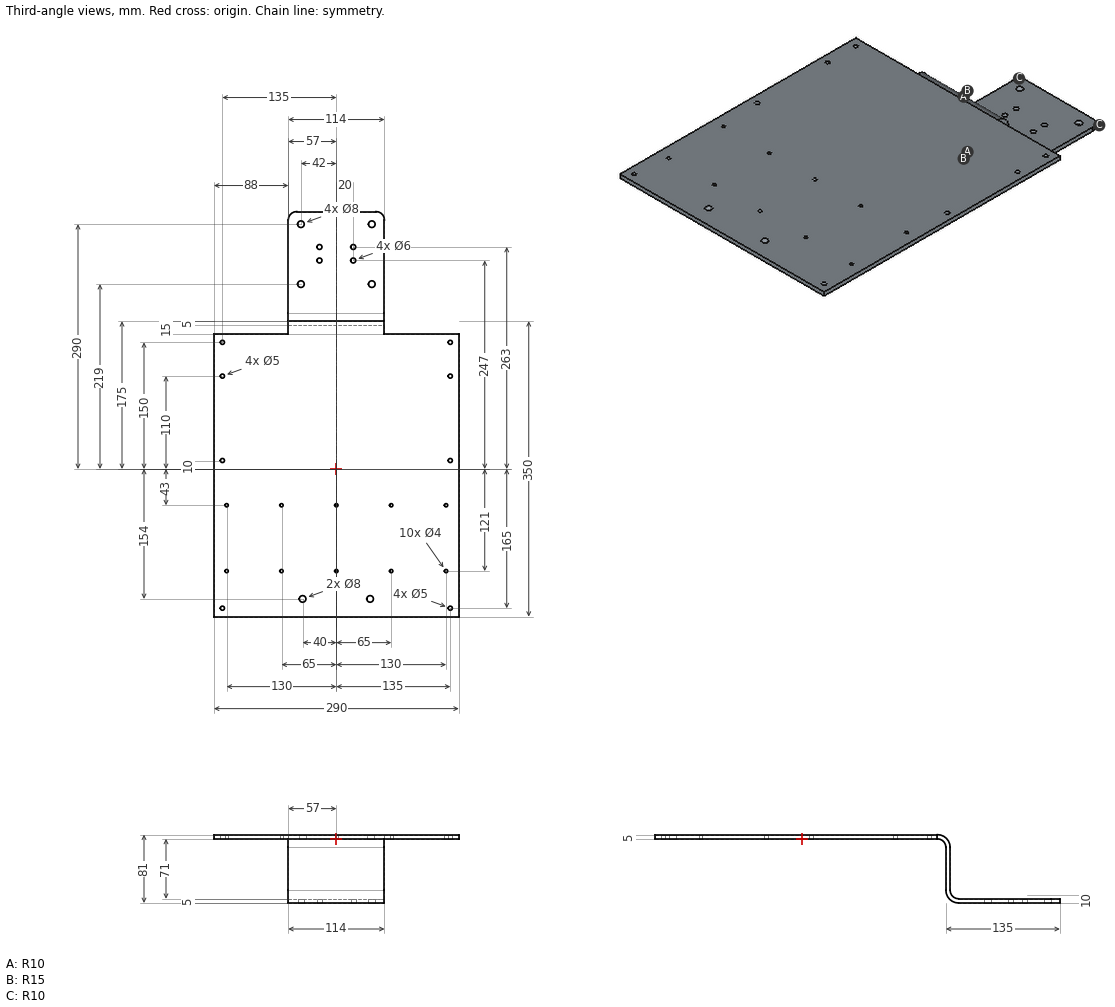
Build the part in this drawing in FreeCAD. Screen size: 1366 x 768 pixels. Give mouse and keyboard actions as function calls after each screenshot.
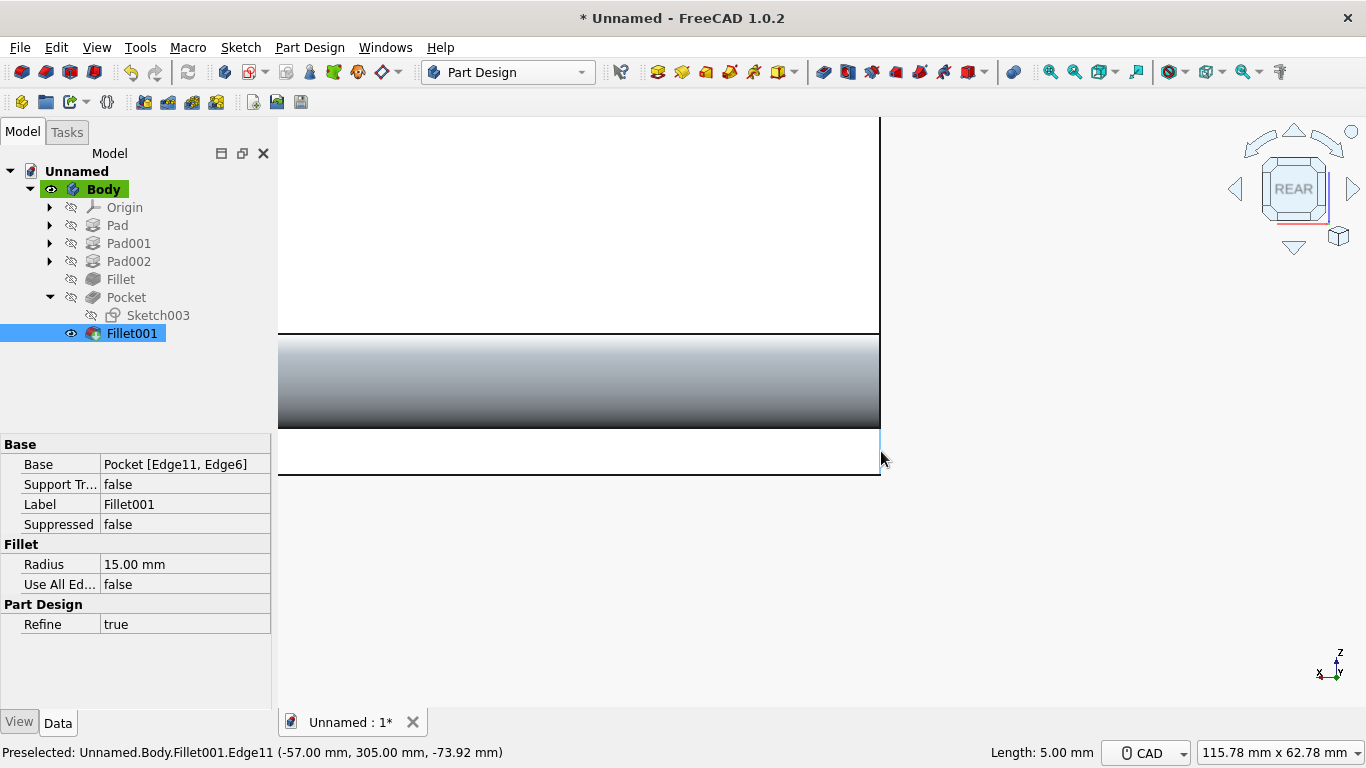
click(880, 451, ctrl)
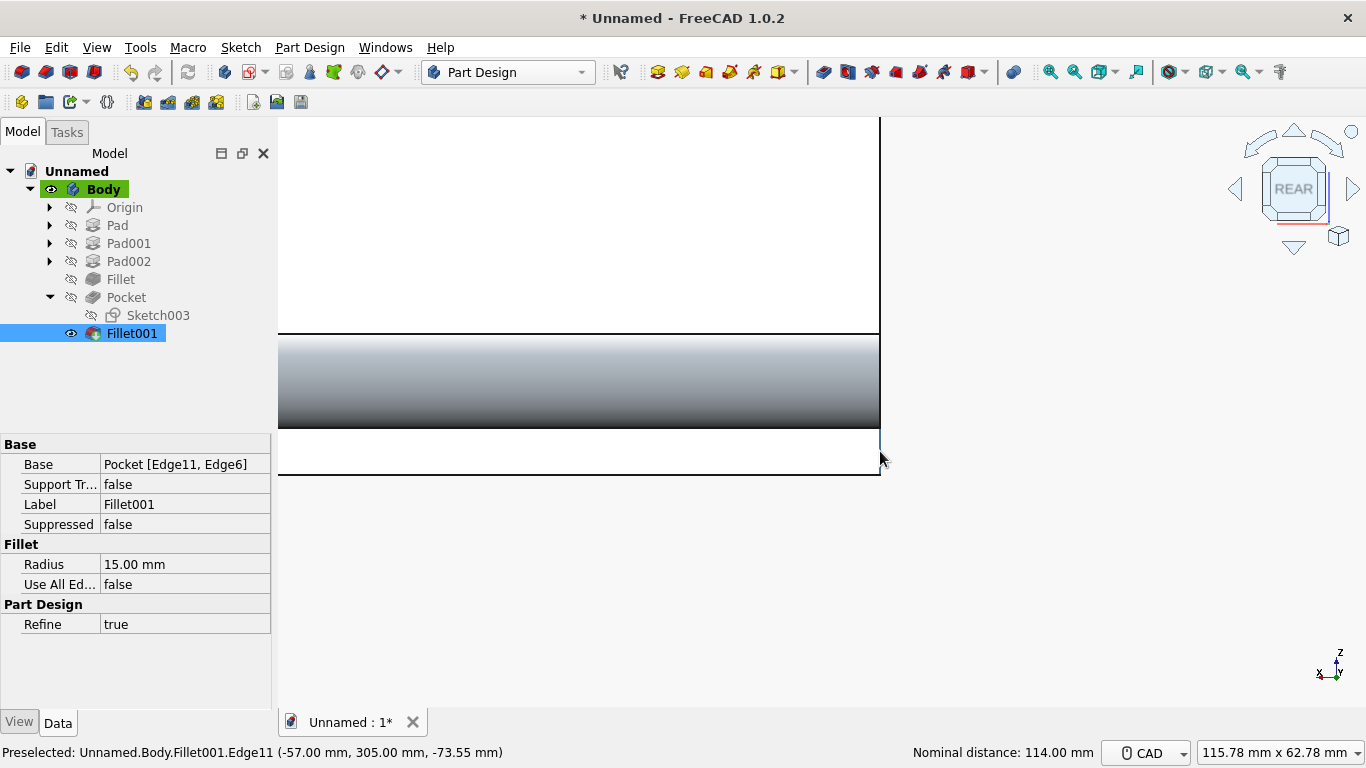
click(22, 72)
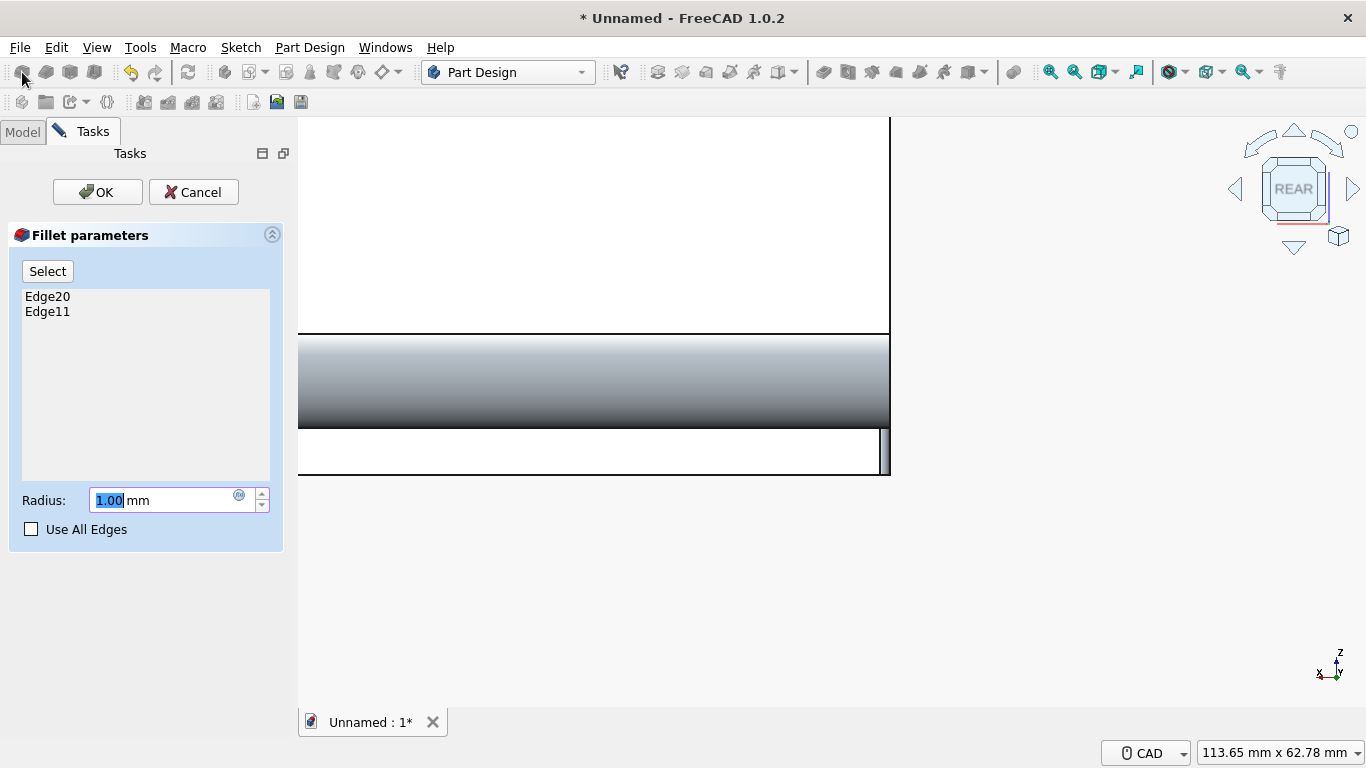
text(10)
key(Tab)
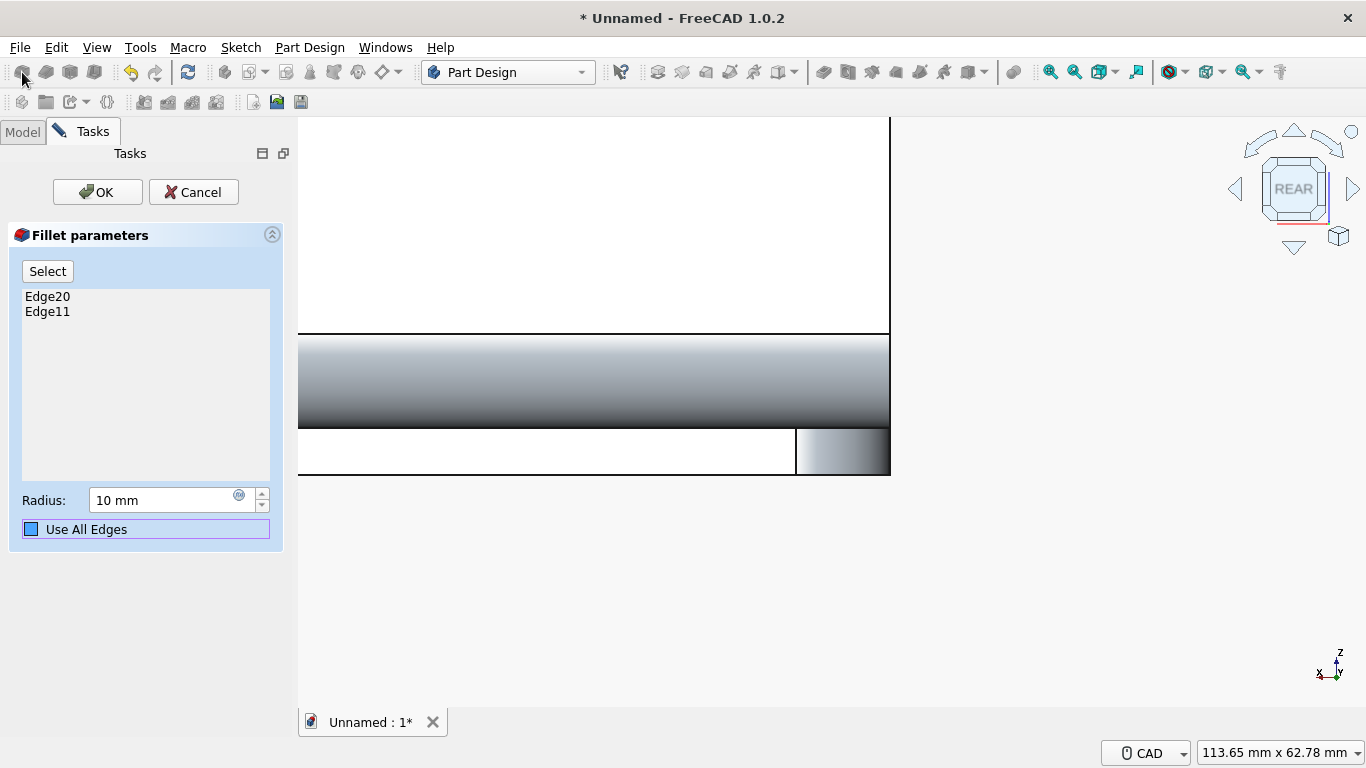
click(98, 192)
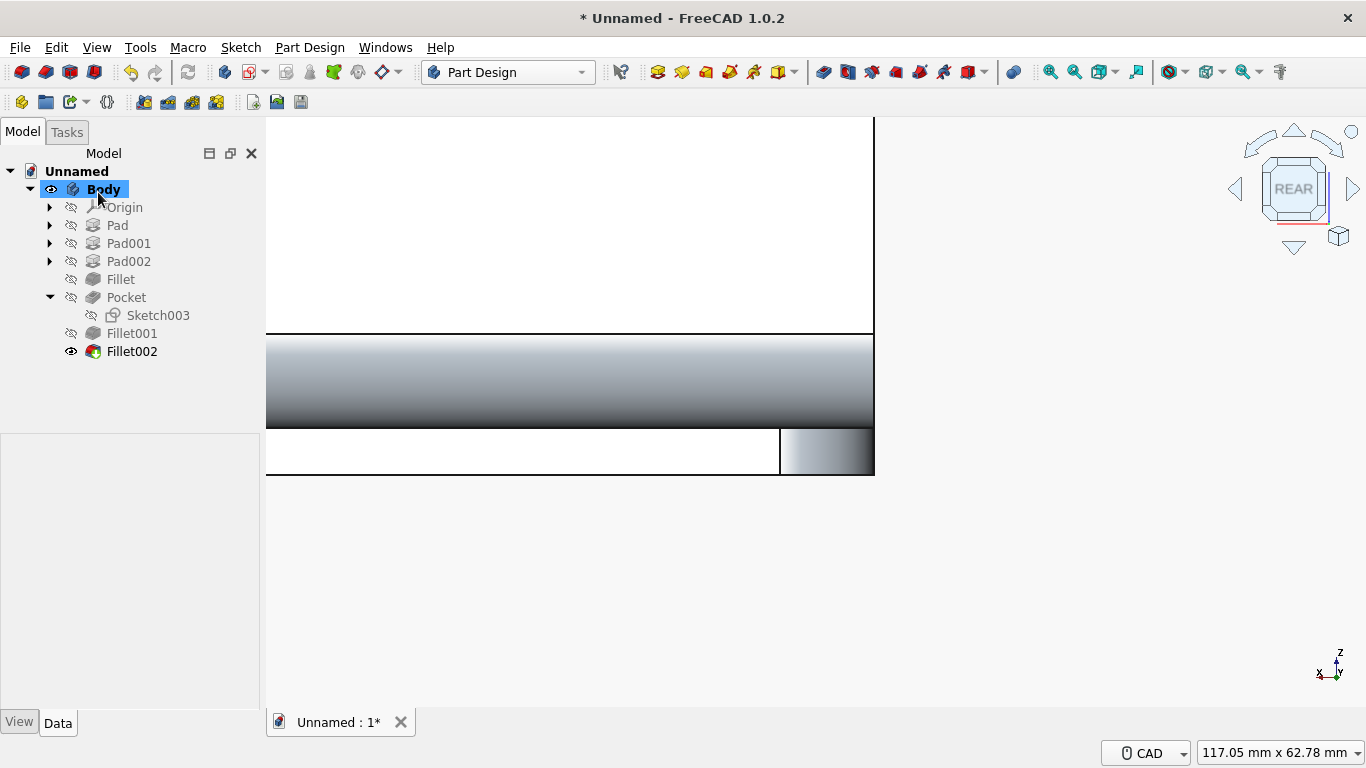
click(1052, 72)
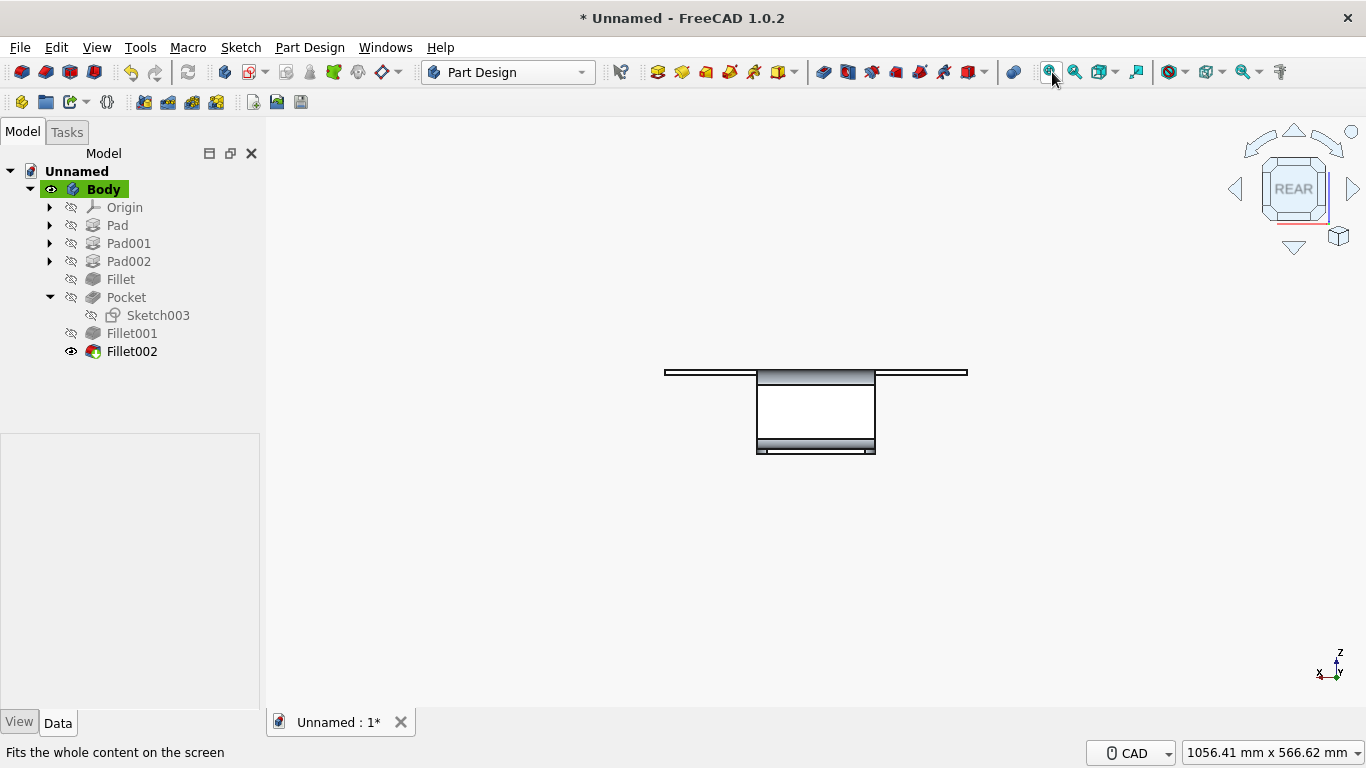
key(5)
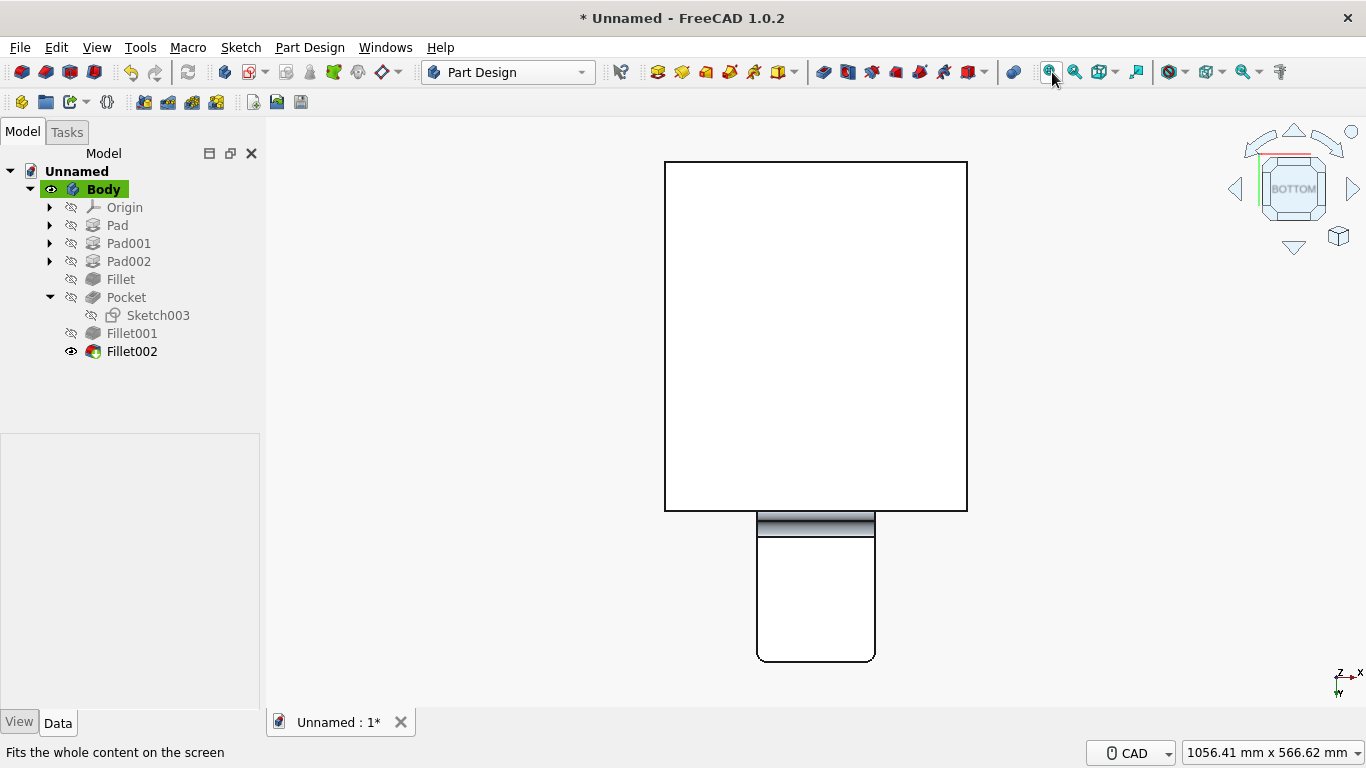
click(816, 598)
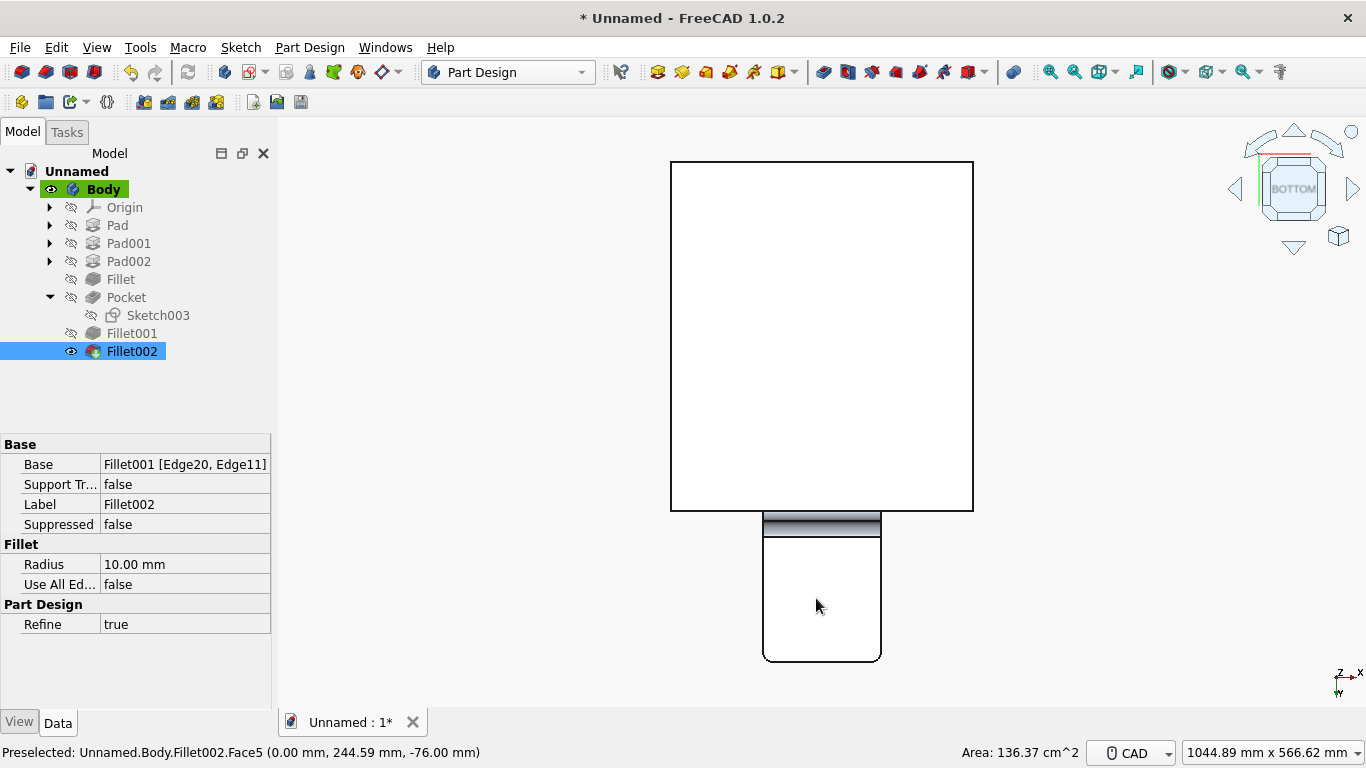
click(250, 72)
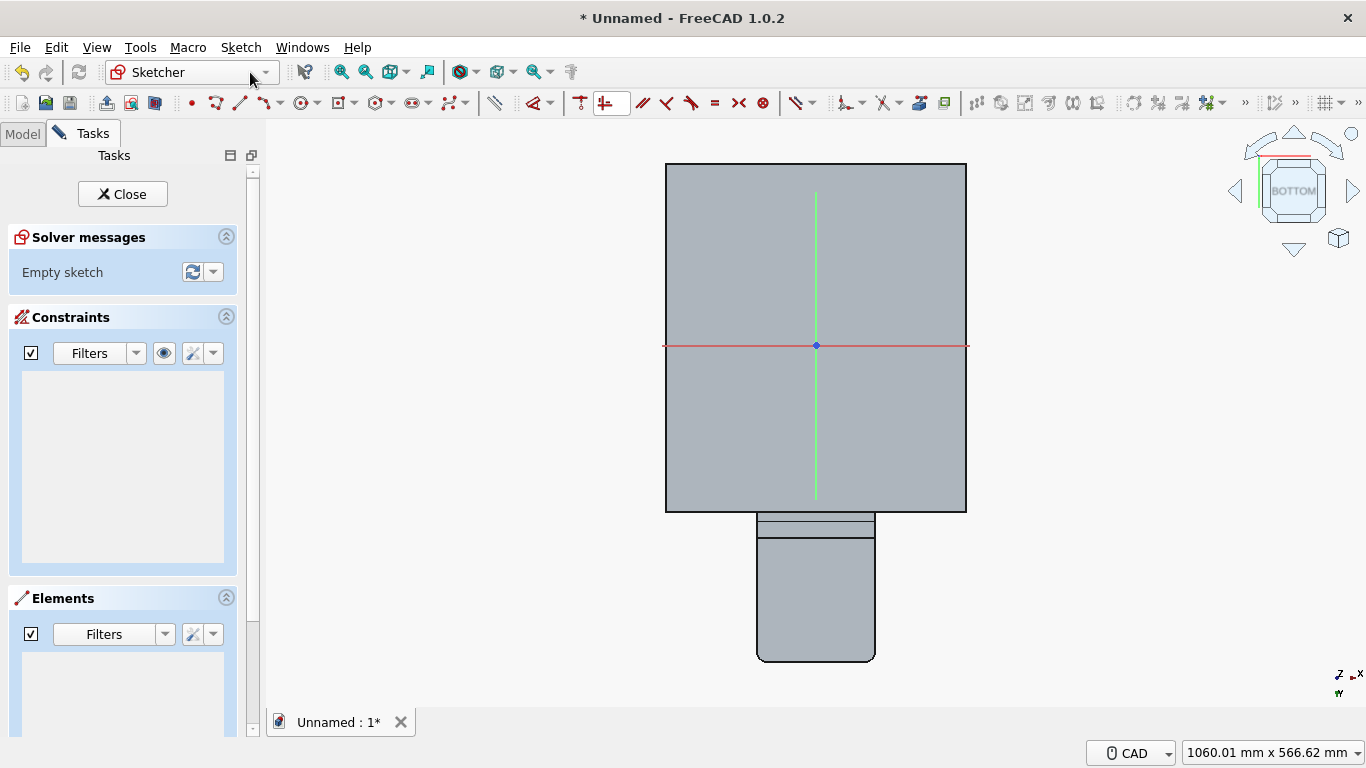
scroll(833, 659, up, 8)